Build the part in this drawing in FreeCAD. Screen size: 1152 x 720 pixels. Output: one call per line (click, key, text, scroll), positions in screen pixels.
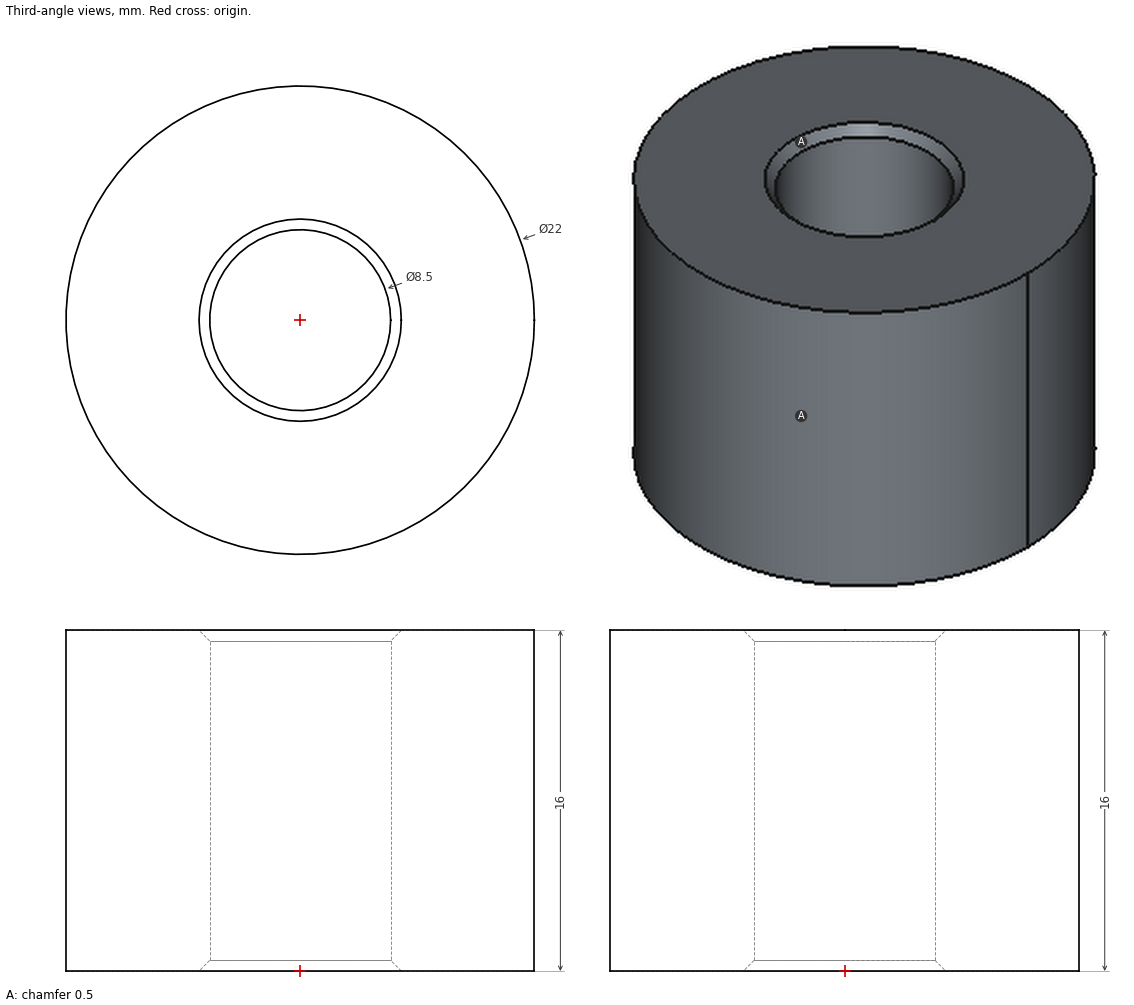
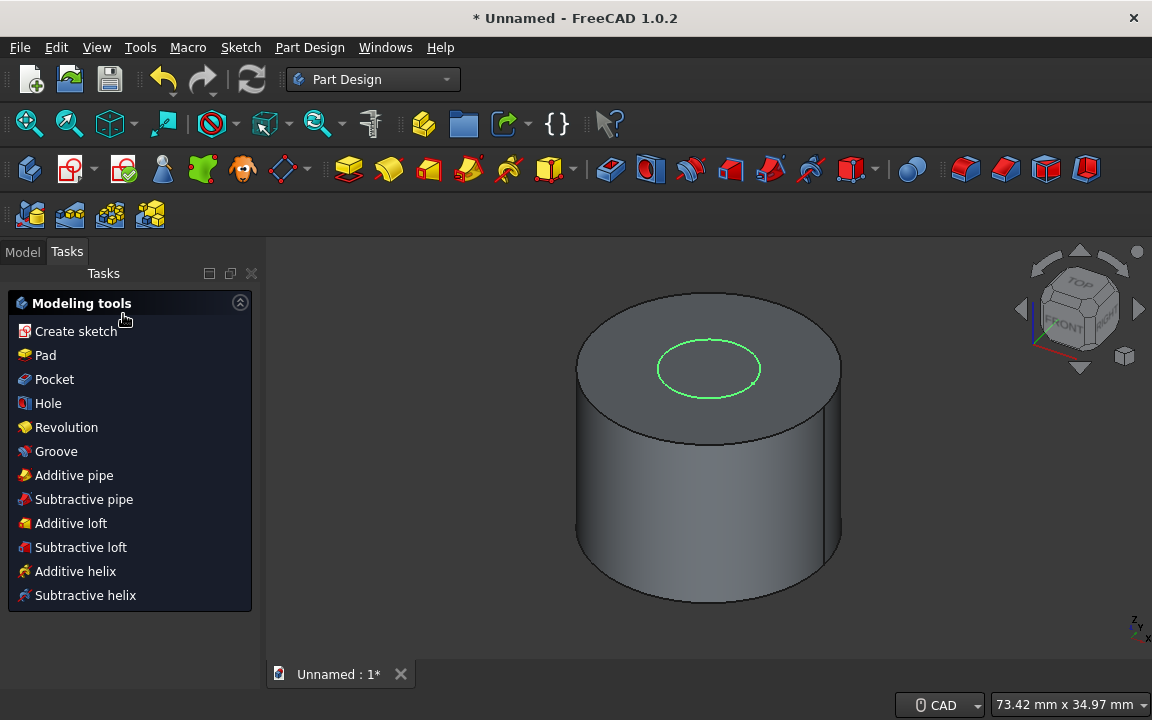
click(612, 170)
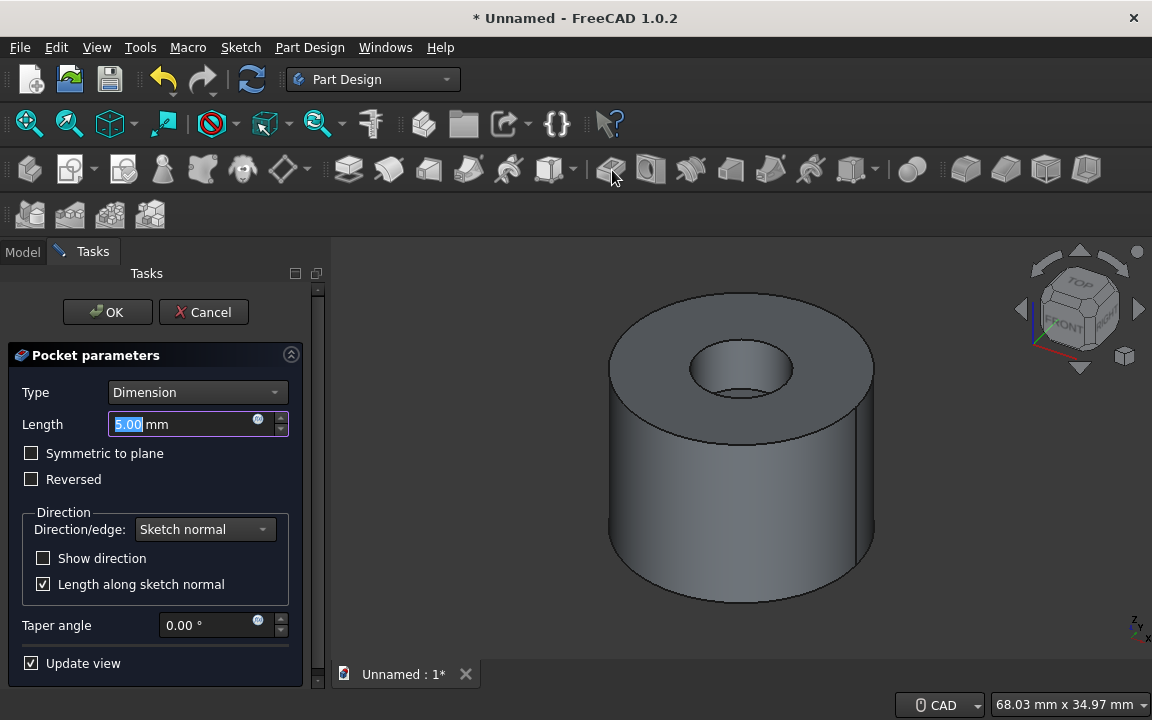
text(16)
key(Tab)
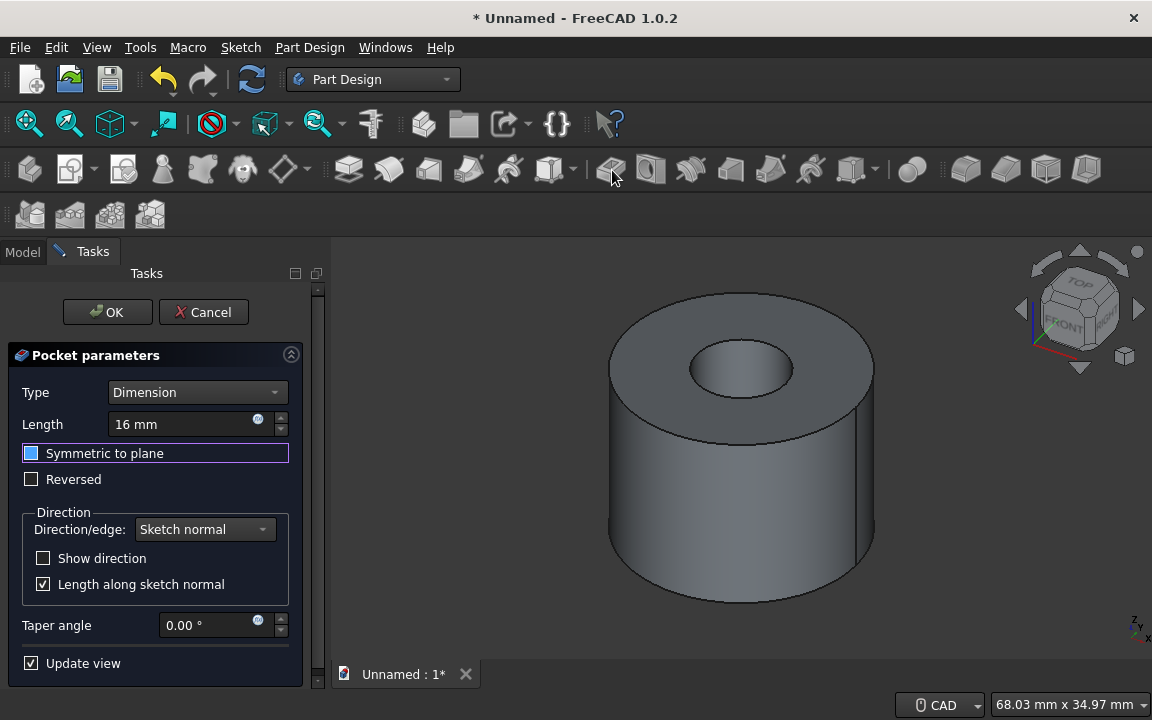
click(108, 312)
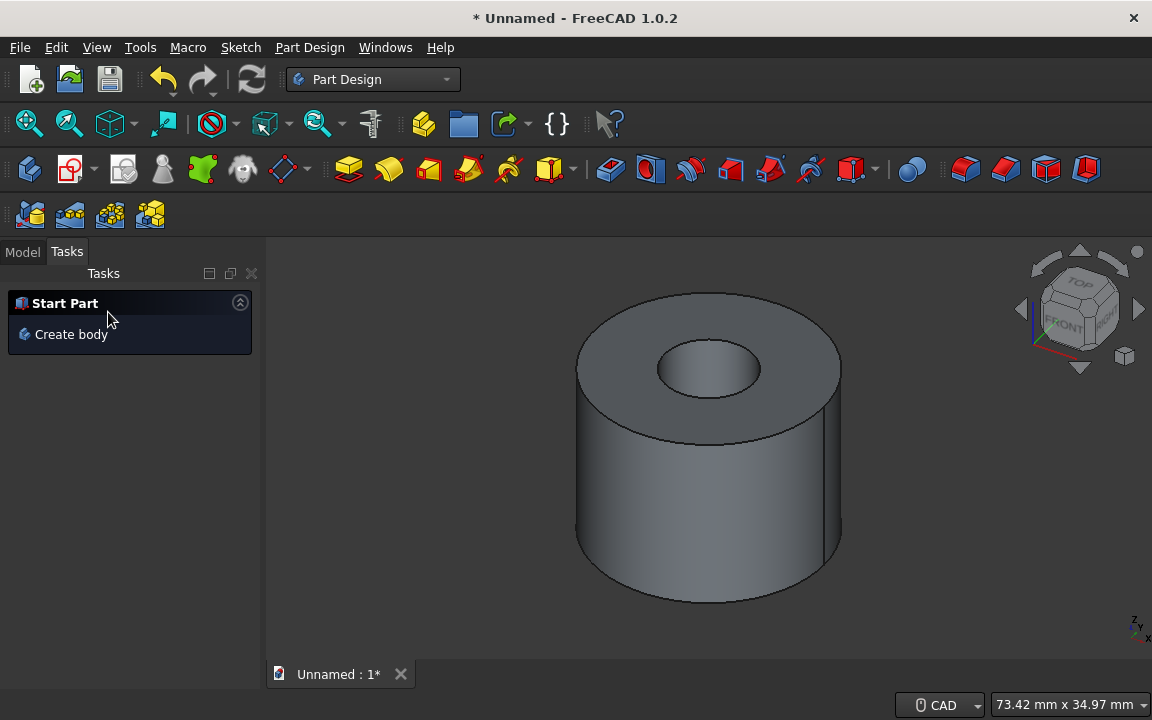
click(664, 353)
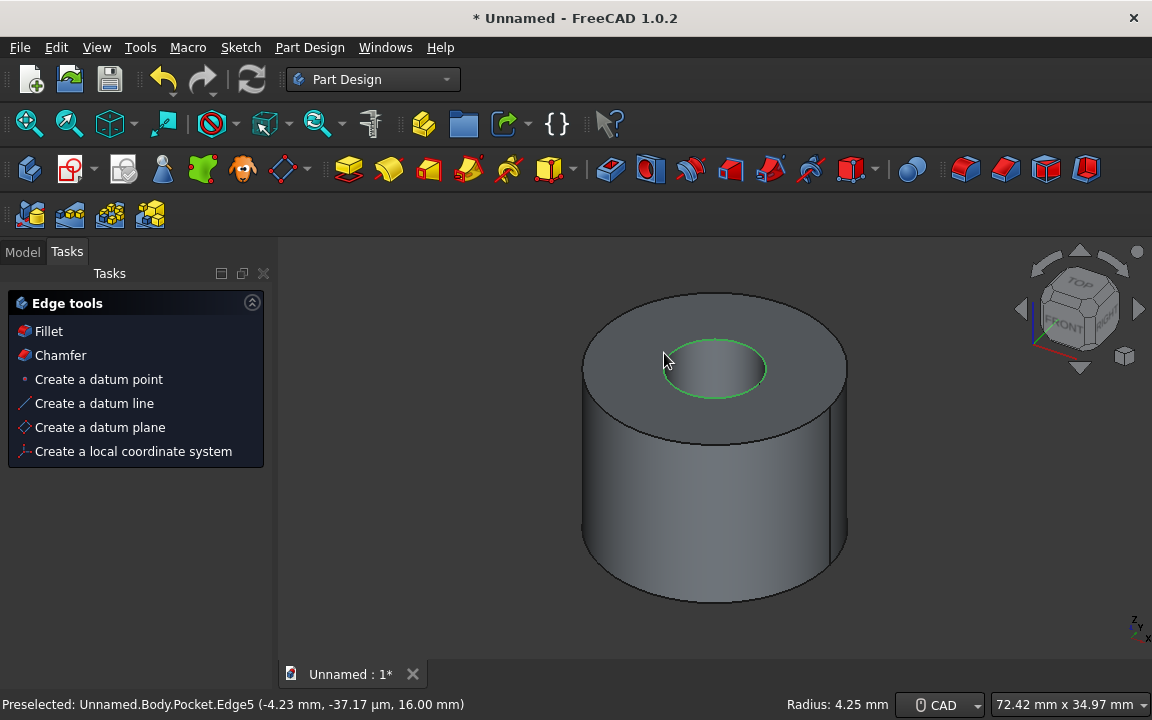
key(0)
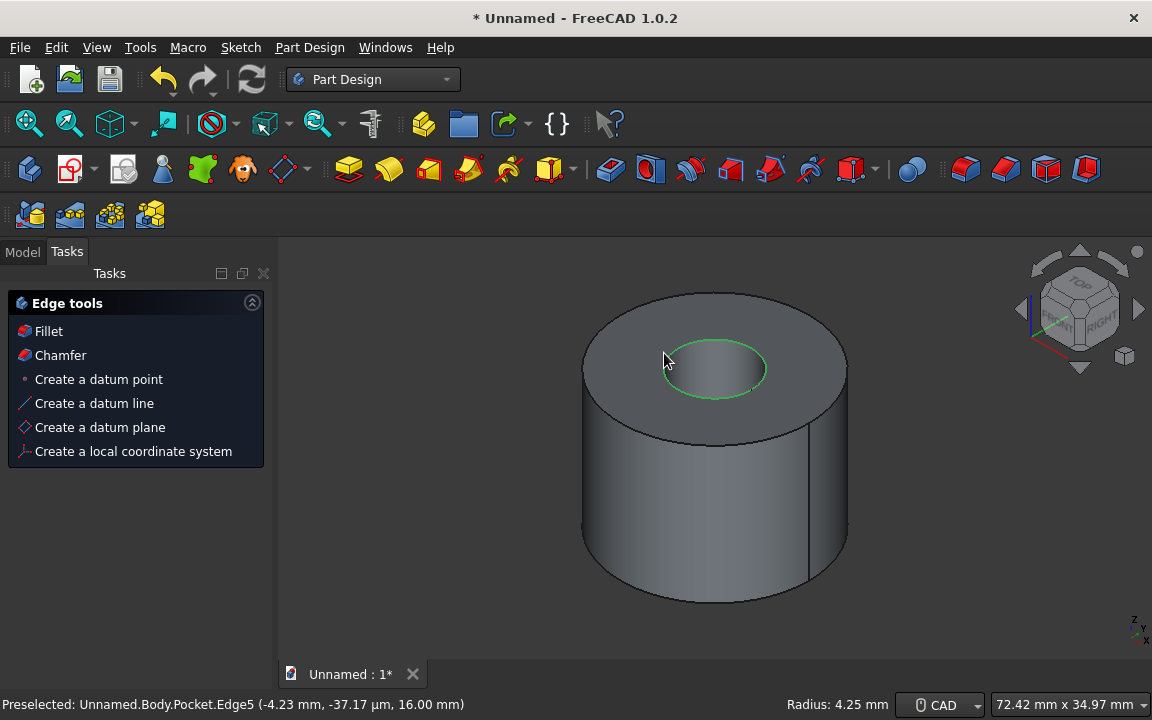
key(2)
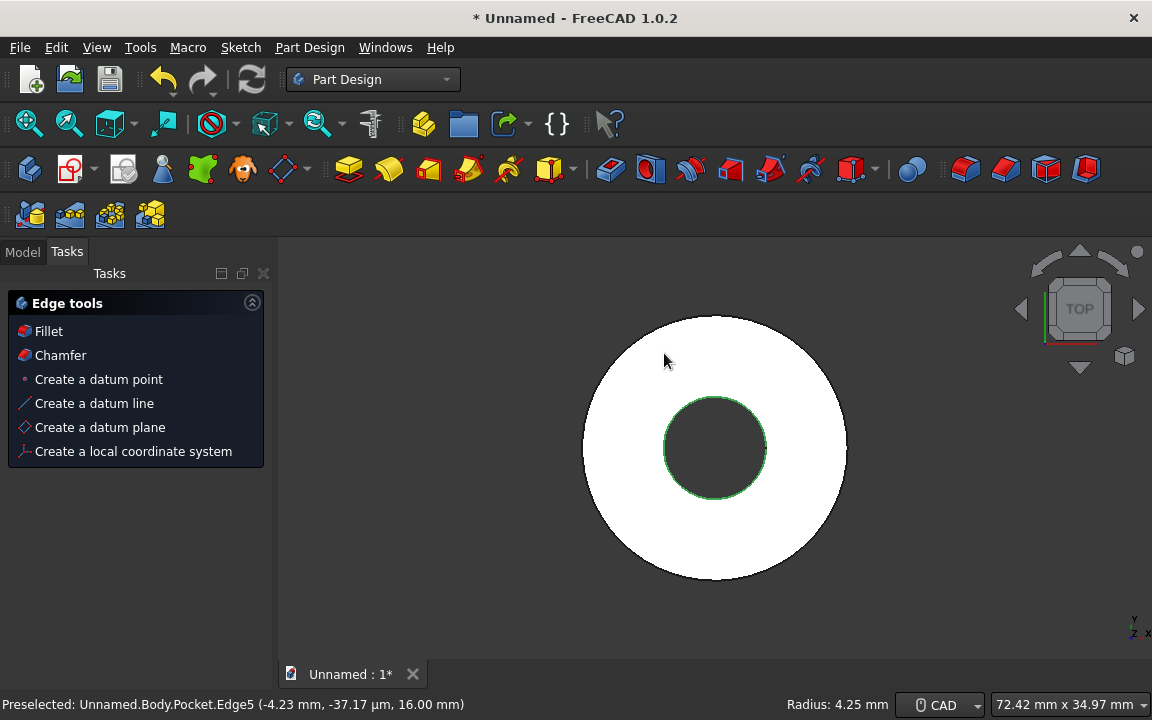
key(1)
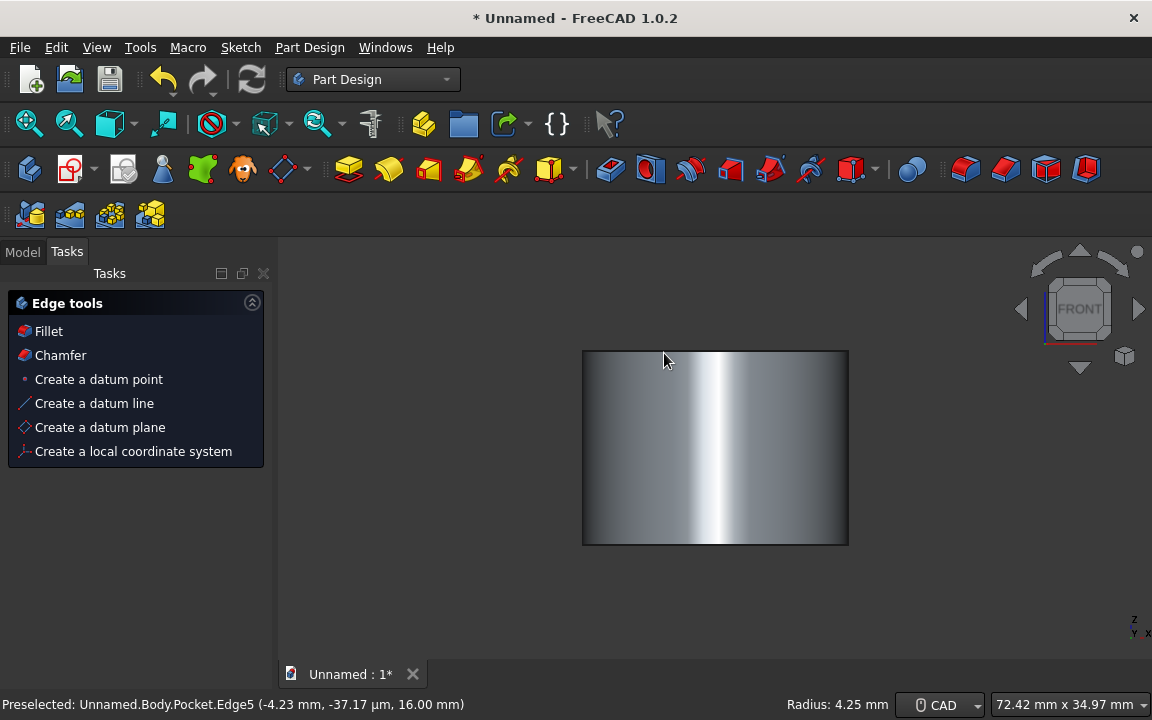
key(3)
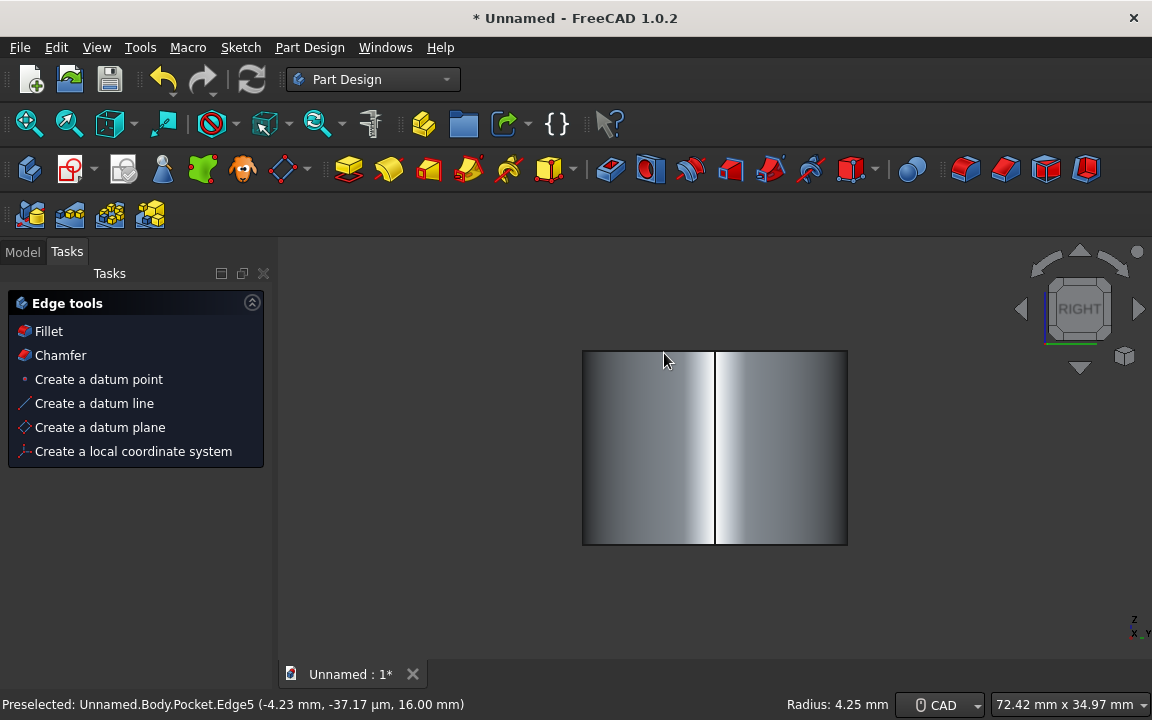
key(5)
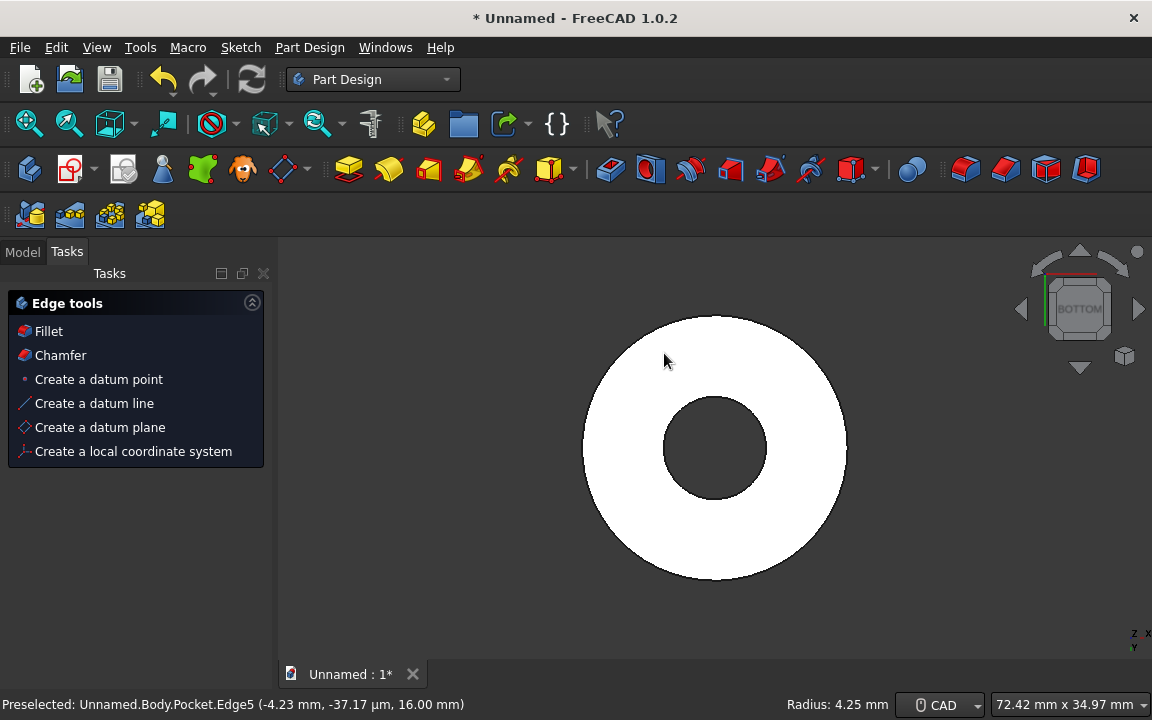
click(664, 447, ctrl)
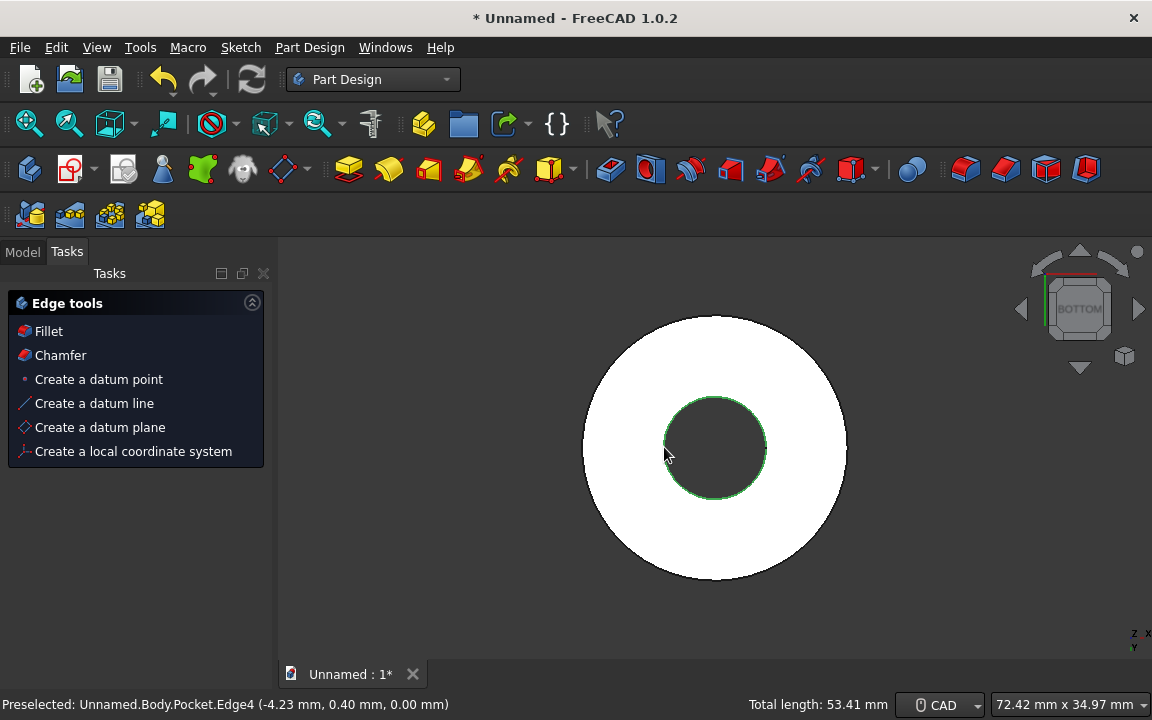
click(1006, 170)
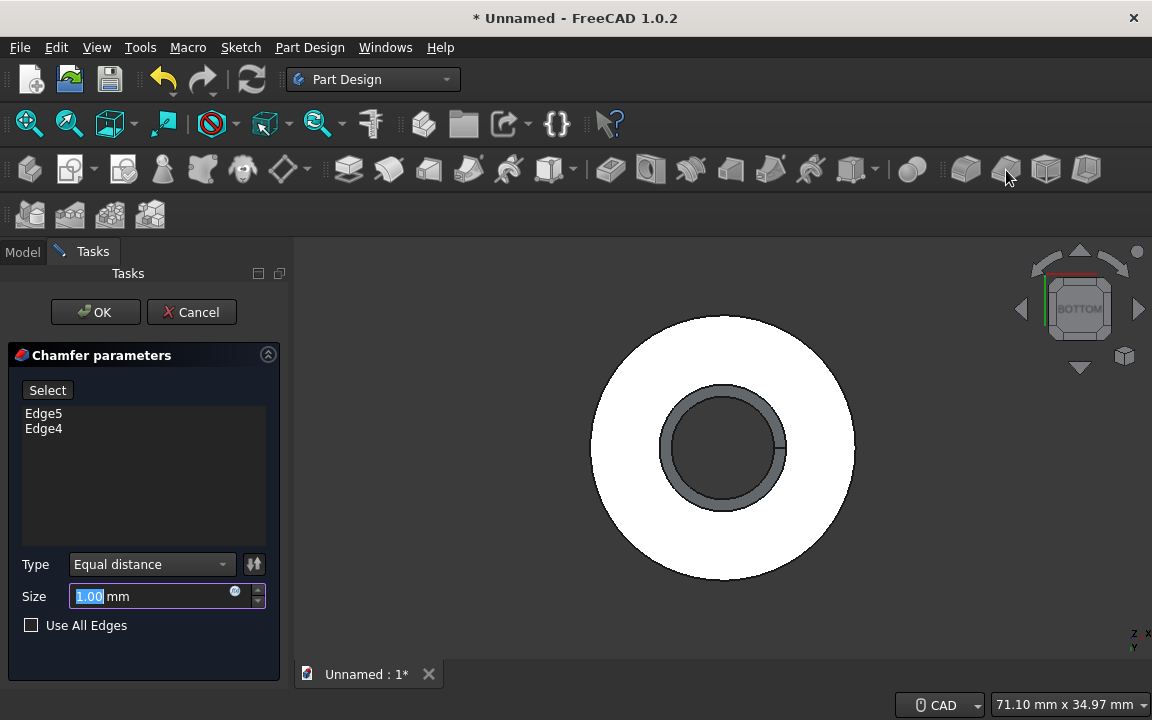
text(0.5)
key(Tab)